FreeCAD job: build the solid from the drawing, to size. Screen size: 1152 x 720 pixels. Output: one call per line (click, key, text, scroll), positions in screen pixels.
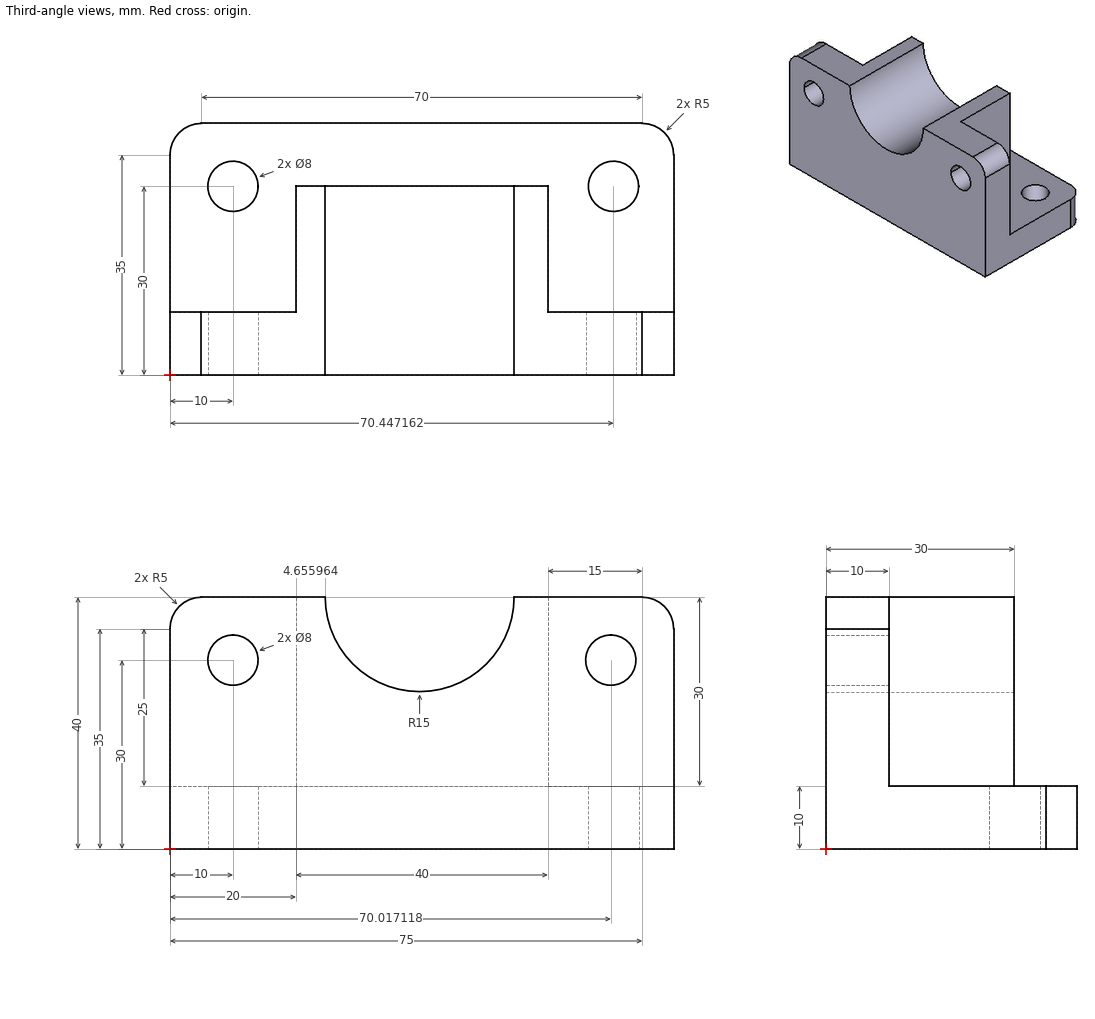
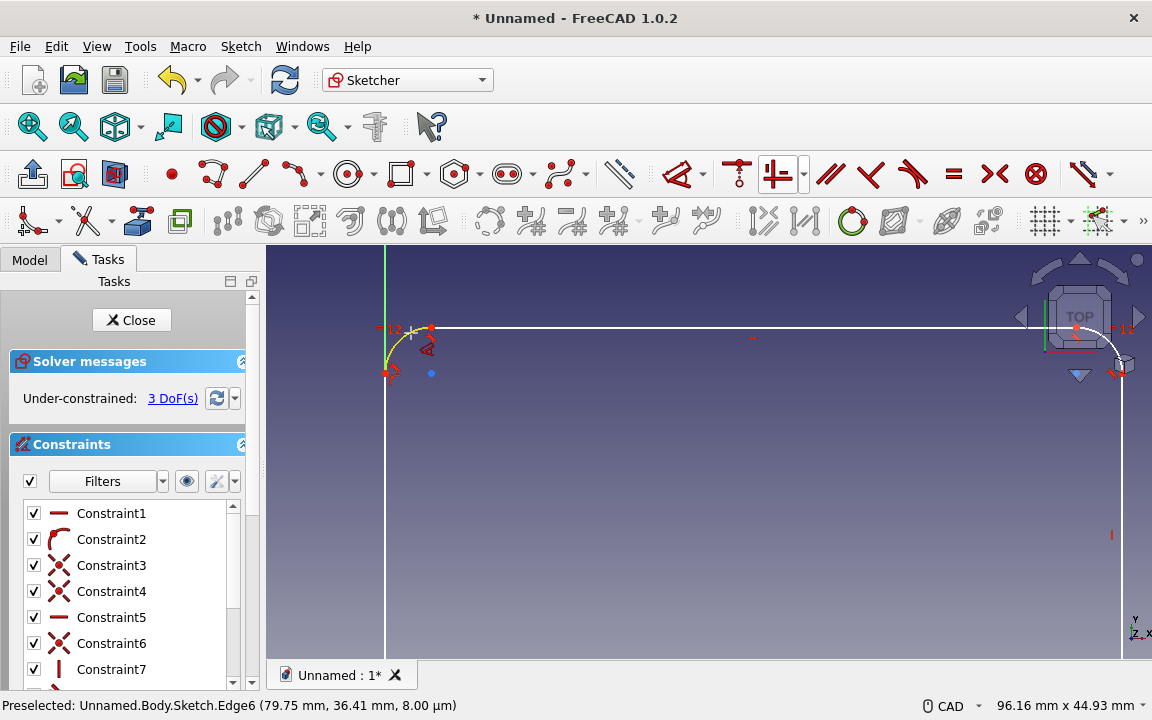
click(411, 333)
click(434, 296)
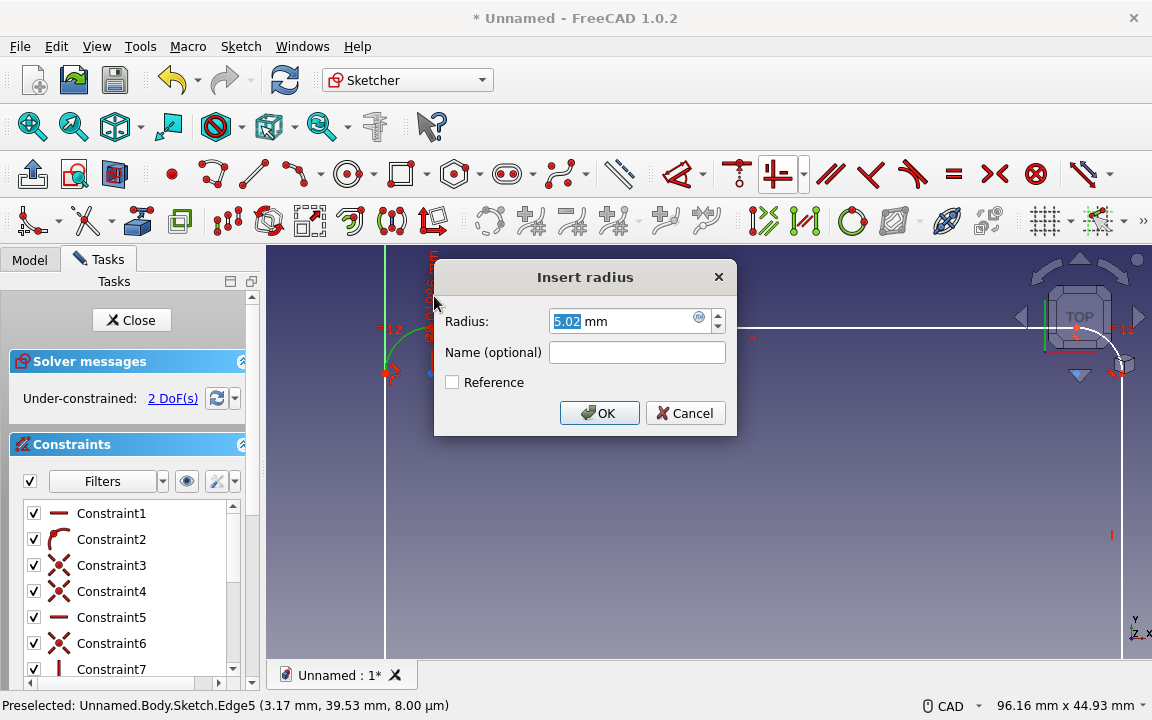
text(5)
key(Return)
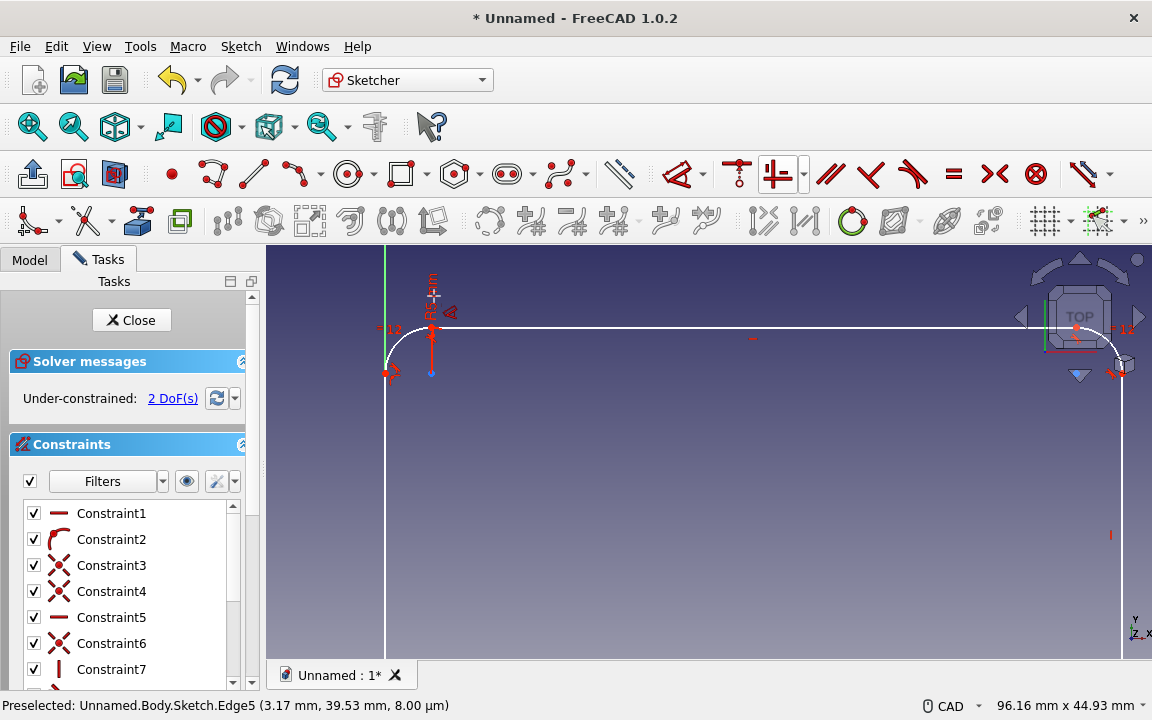
click(883, 328)
click(709, 294)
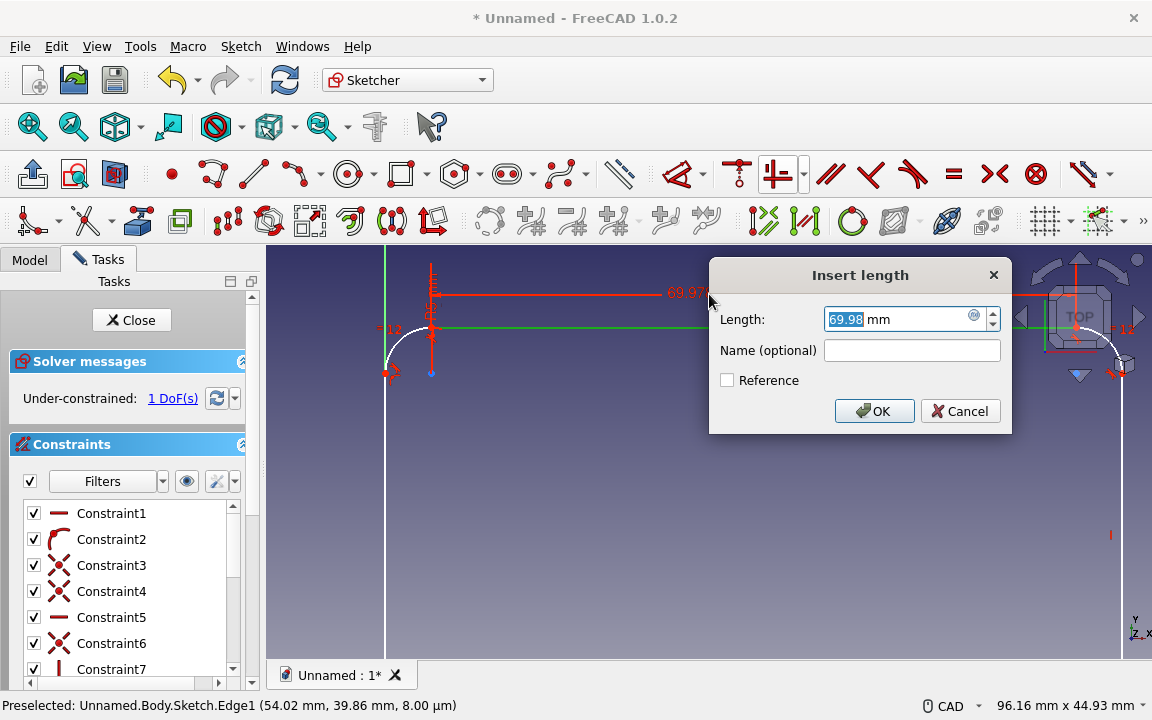
text(70)
key(Return)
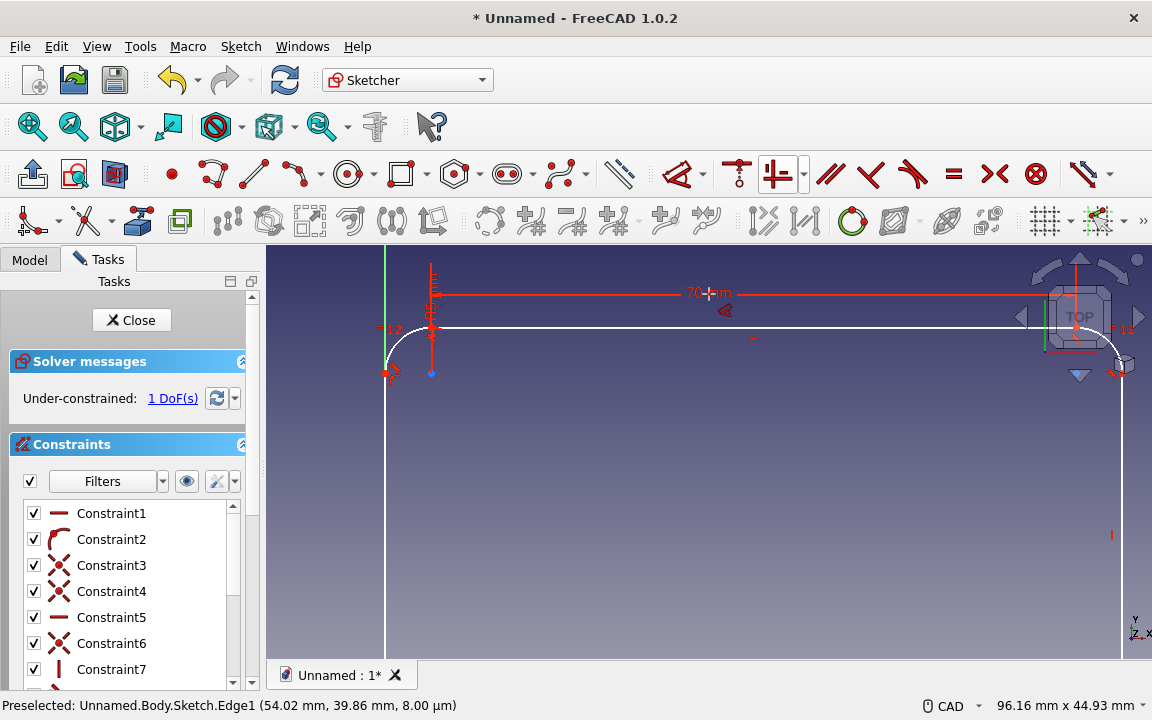
click(385, 470)
click(351, 502)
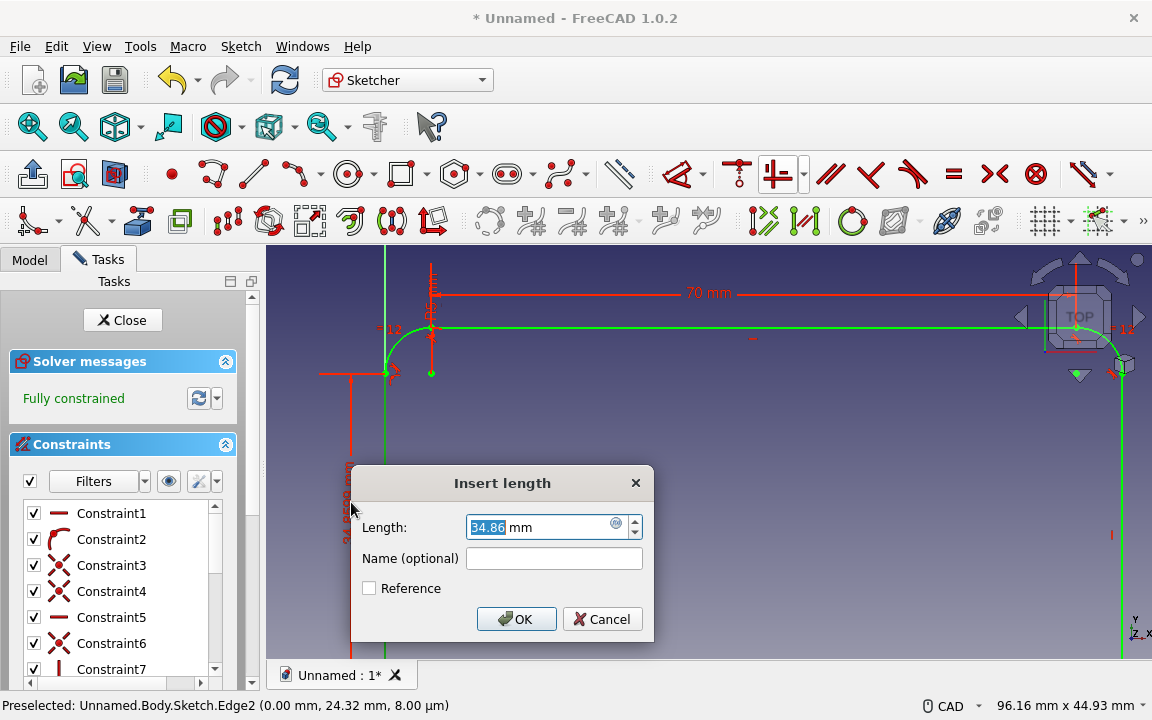
text(35)
key(Return)
key(Escape)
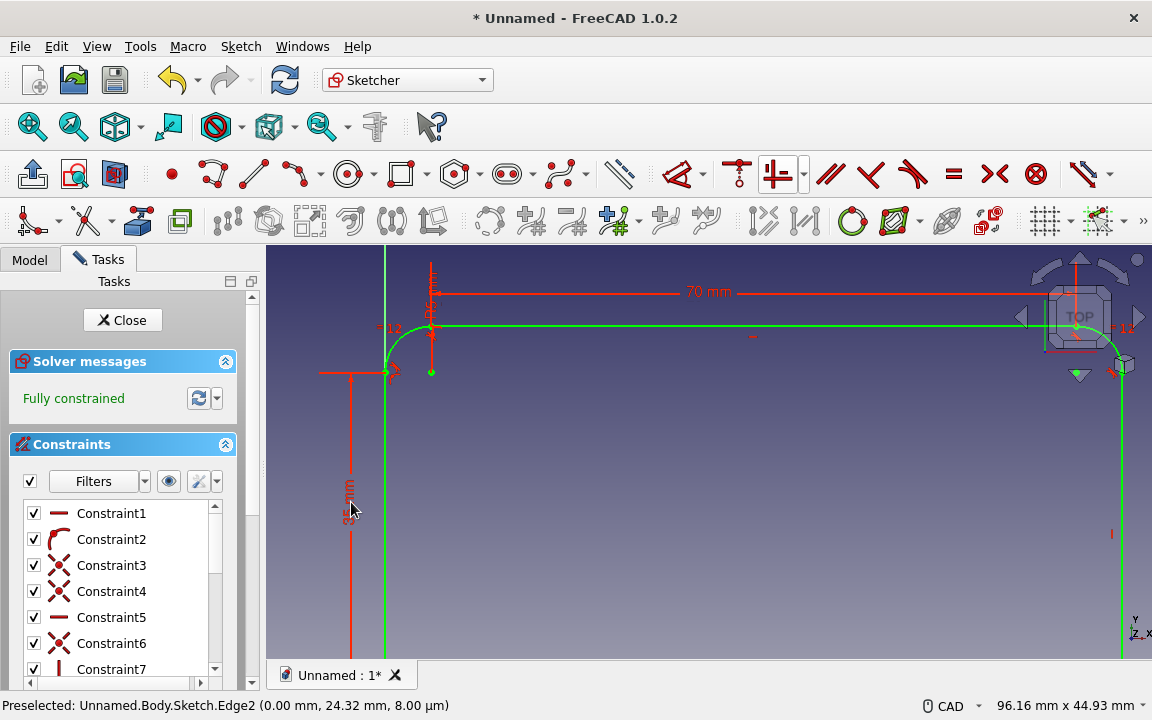
click(123, 320)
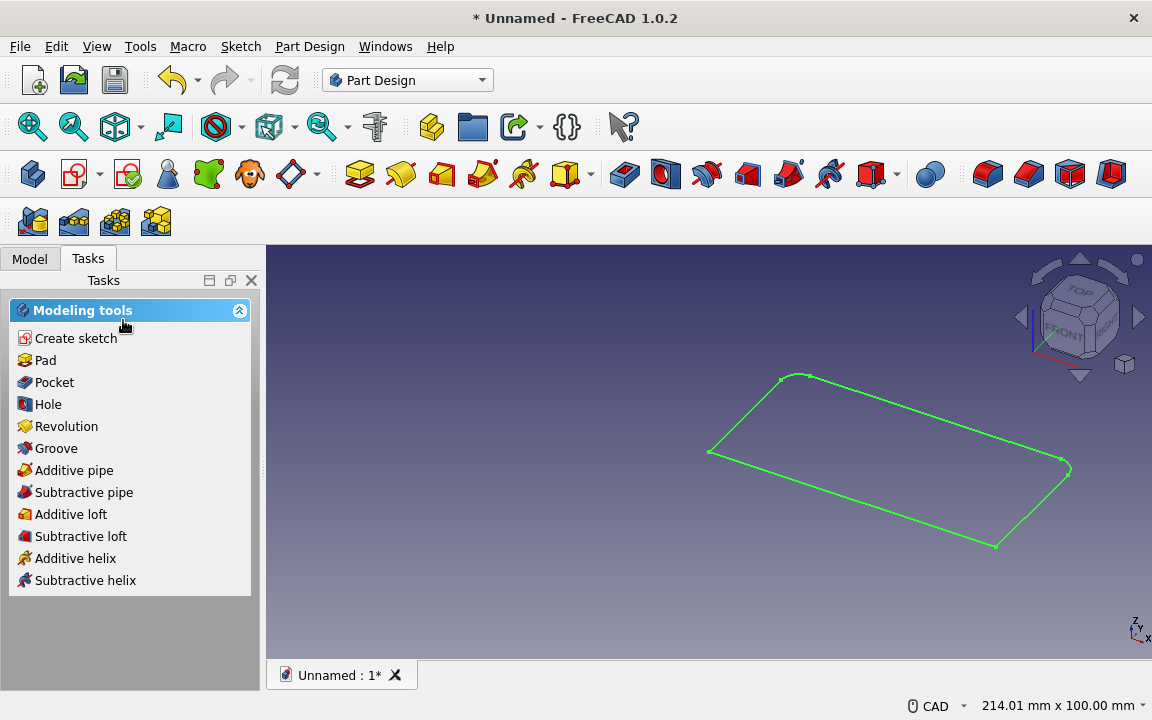
click(360, 174)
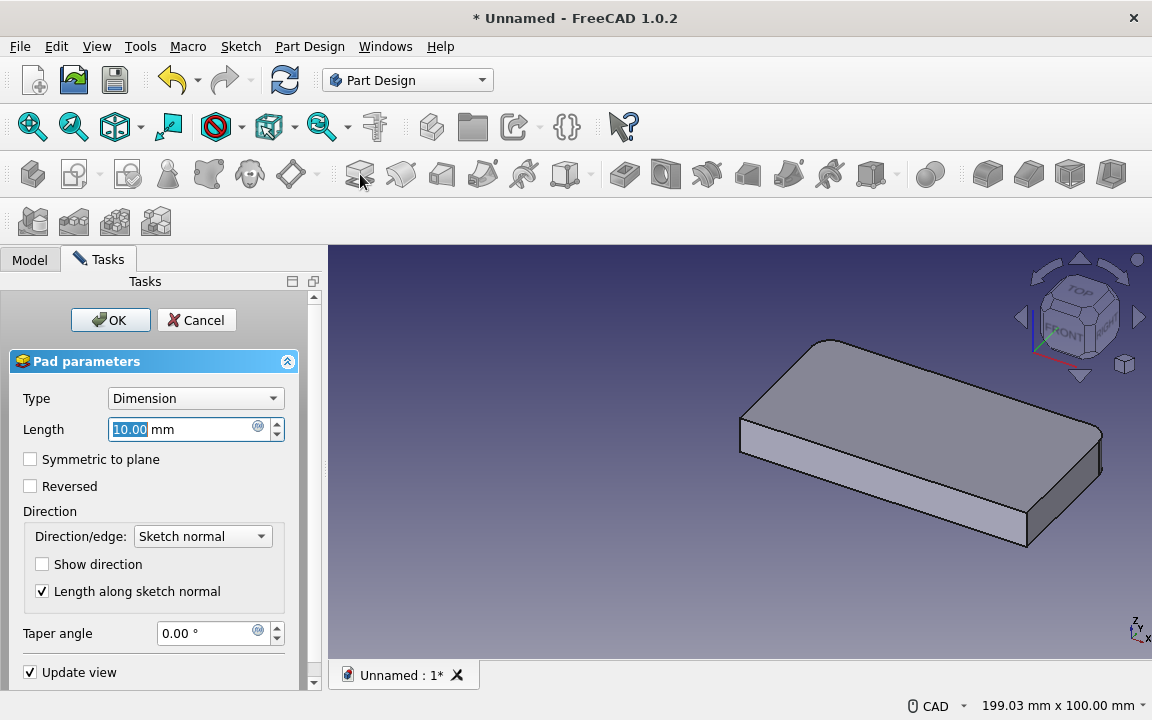
text(10)
key(Tab)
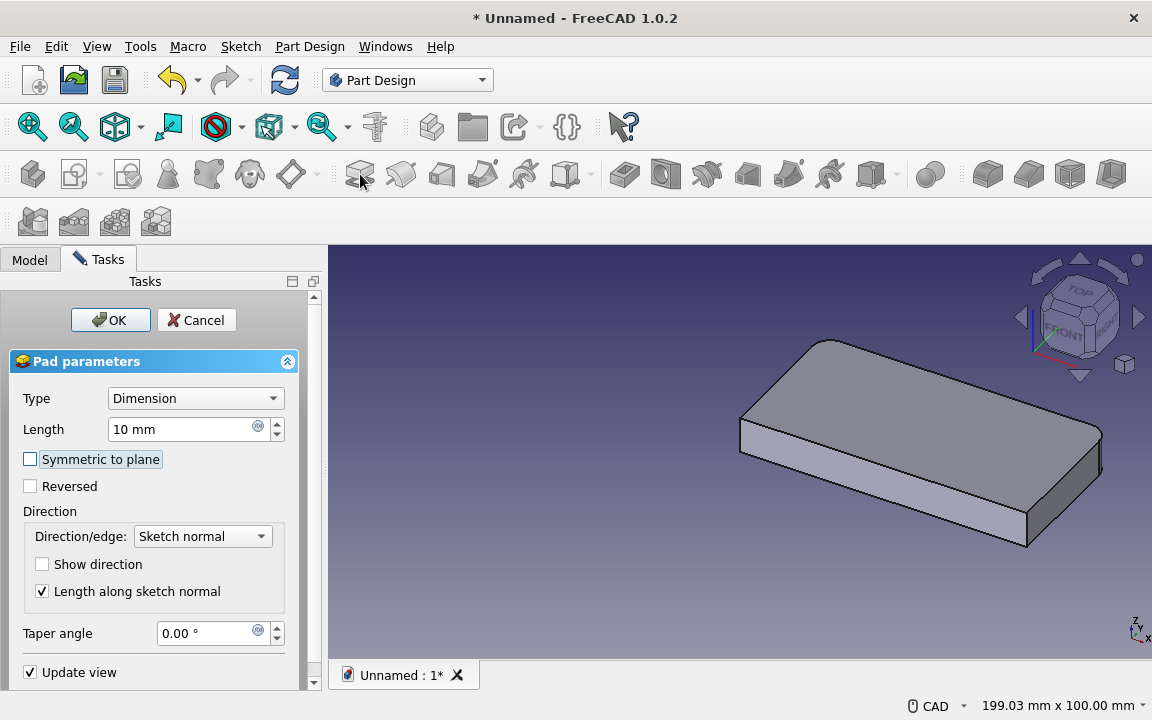
click(111, 320)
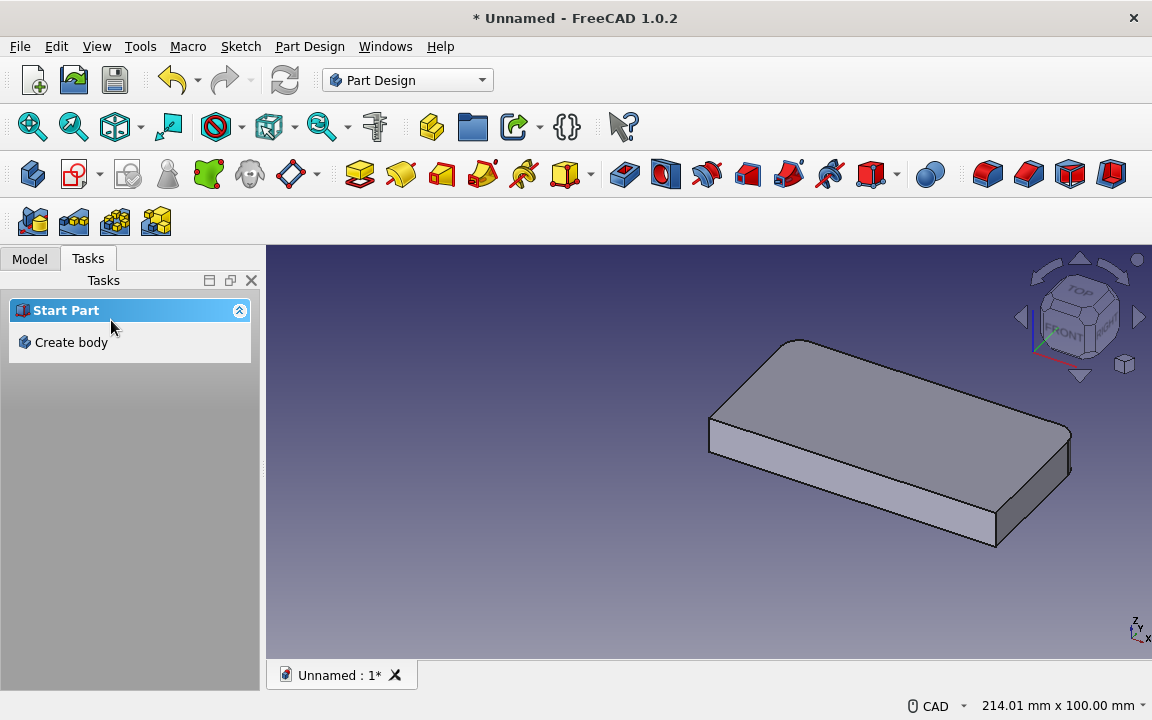
click(975, 522)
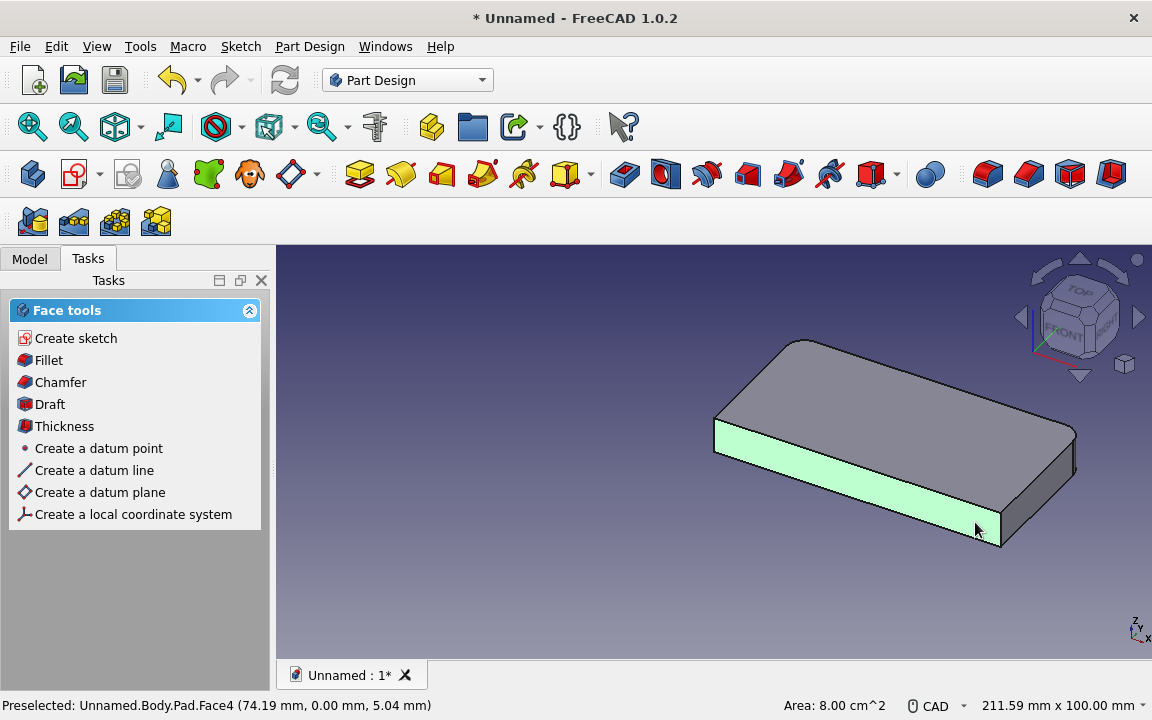
click(74, 174)